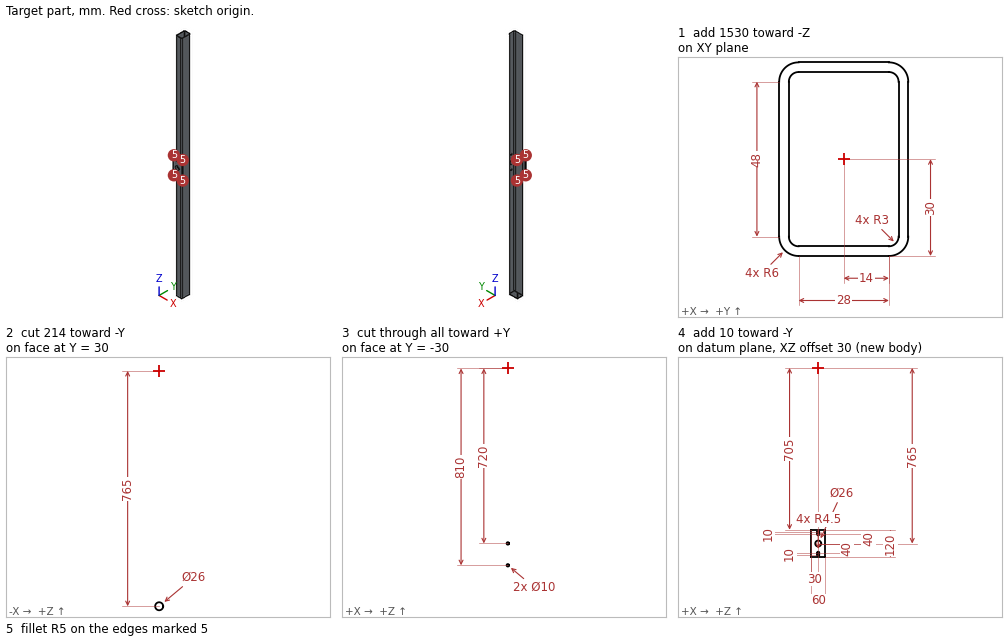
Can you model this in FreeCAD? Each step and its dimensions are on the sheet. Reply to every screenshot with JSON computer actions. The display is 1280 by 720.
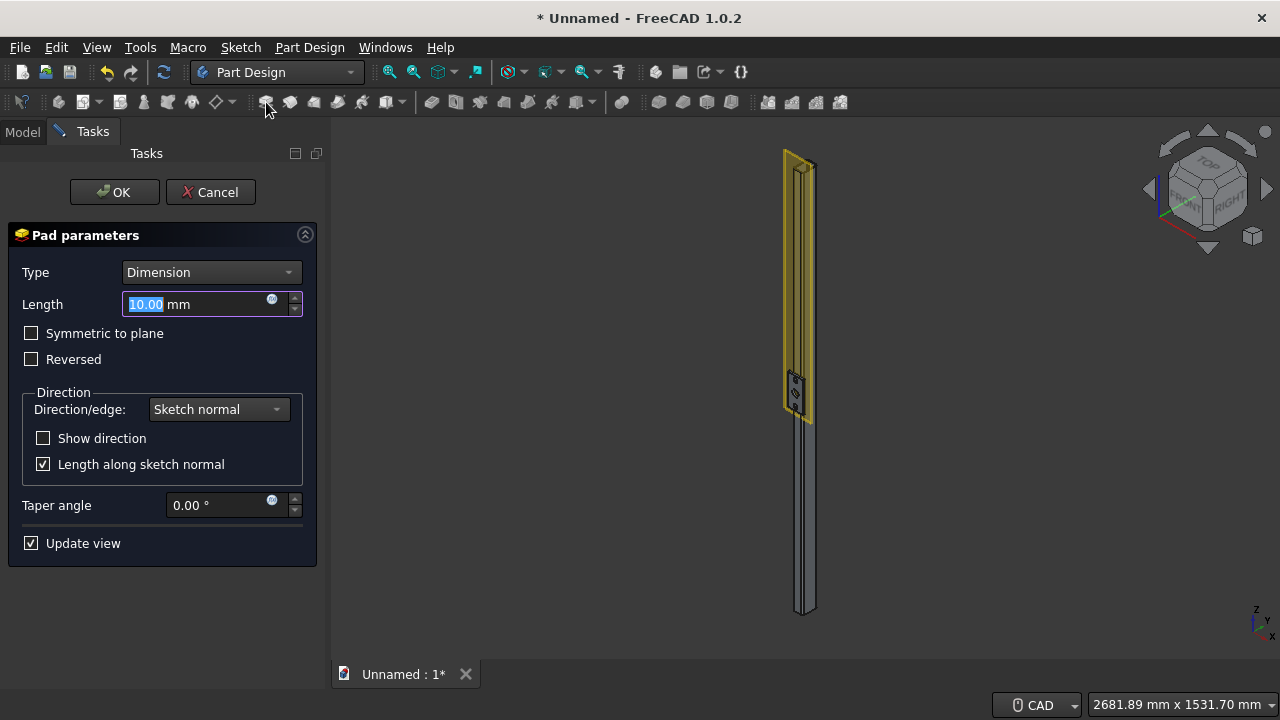
{"action": "type", "text": "10"}
{"action": "key", "text": "Tab"}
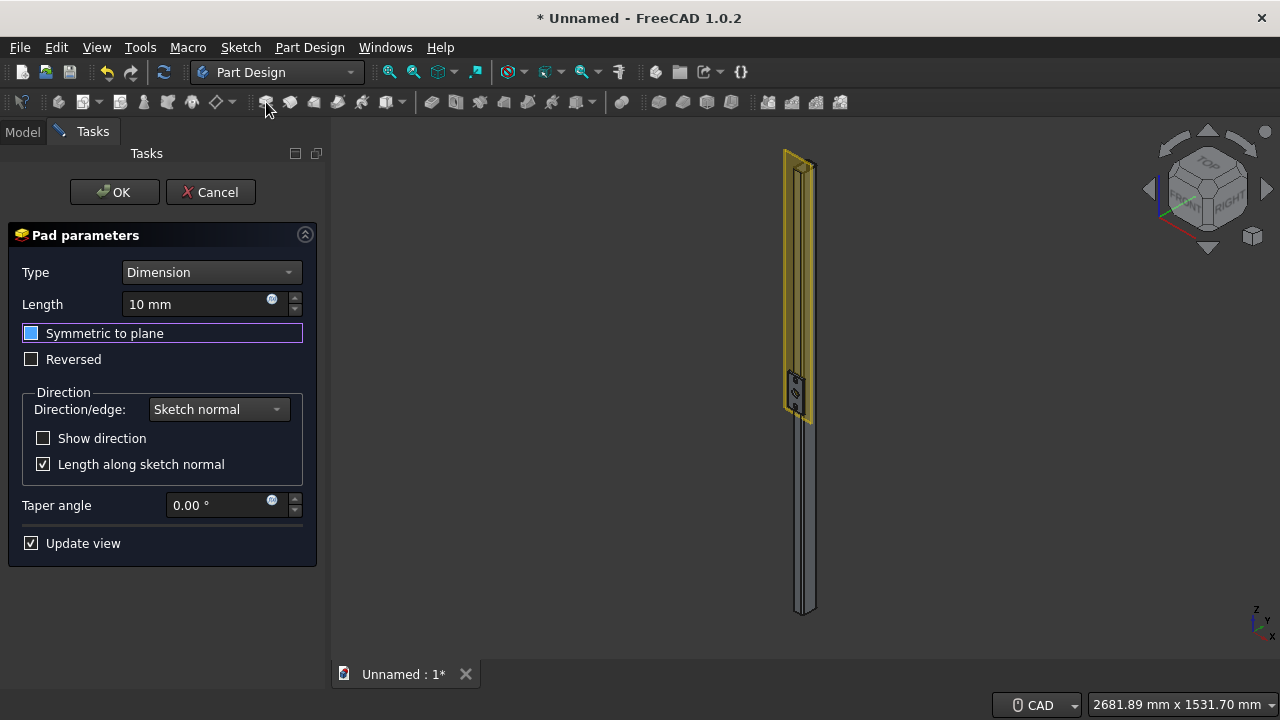
{"action": "left_click", "coordinate": [115, 192]}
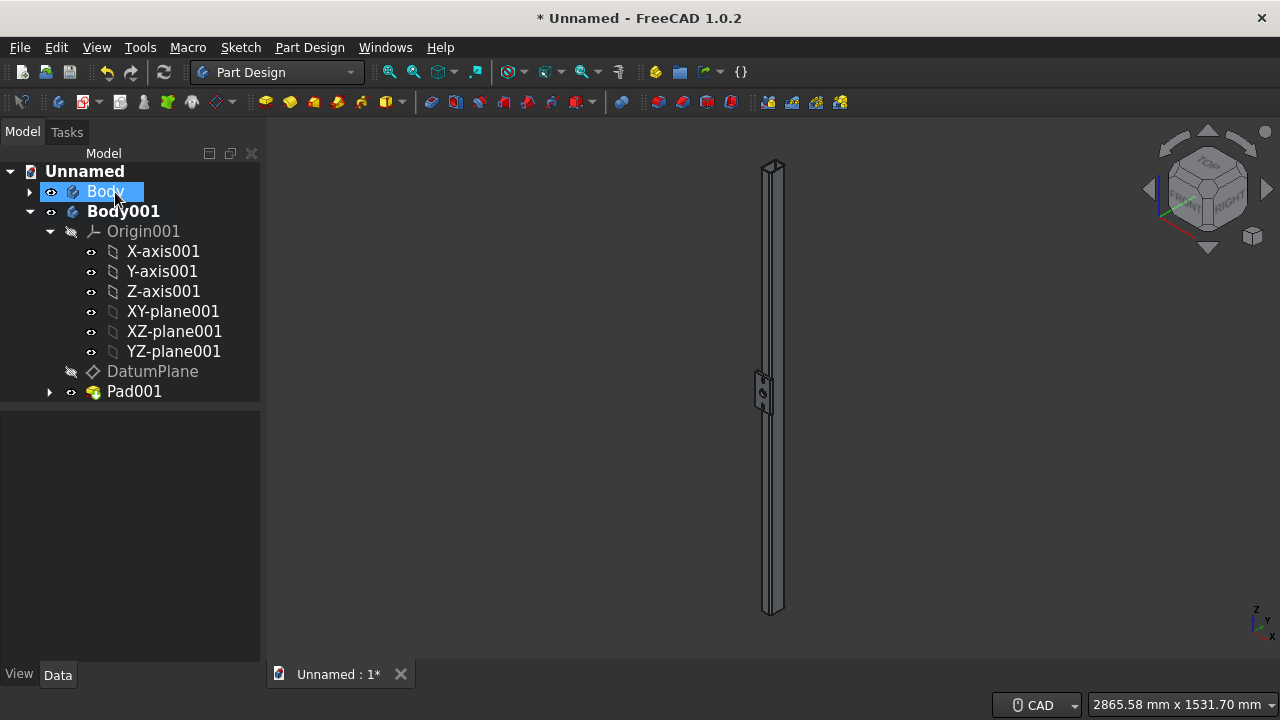
{"action": "left_click", "coordinate": [390, 72]}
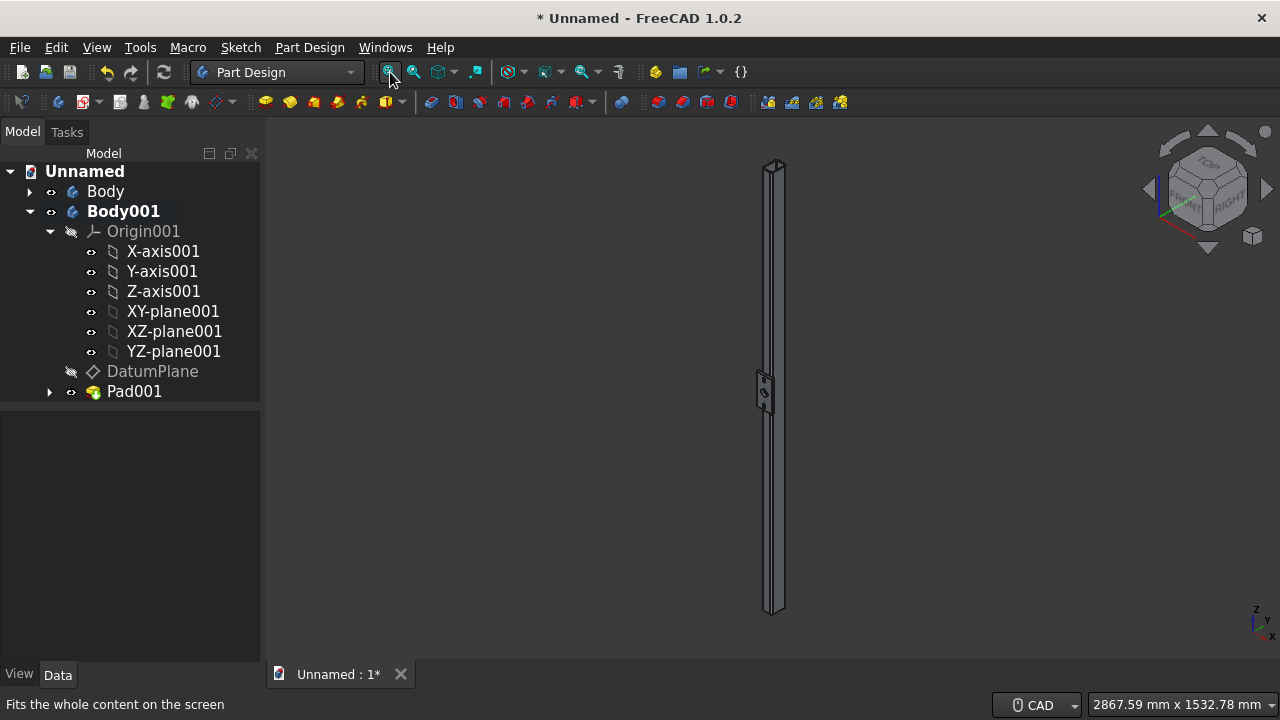
{"action": "scroll", "coordinate": [773, 413], "scroll_direction": "up", "scroll_amount": 13}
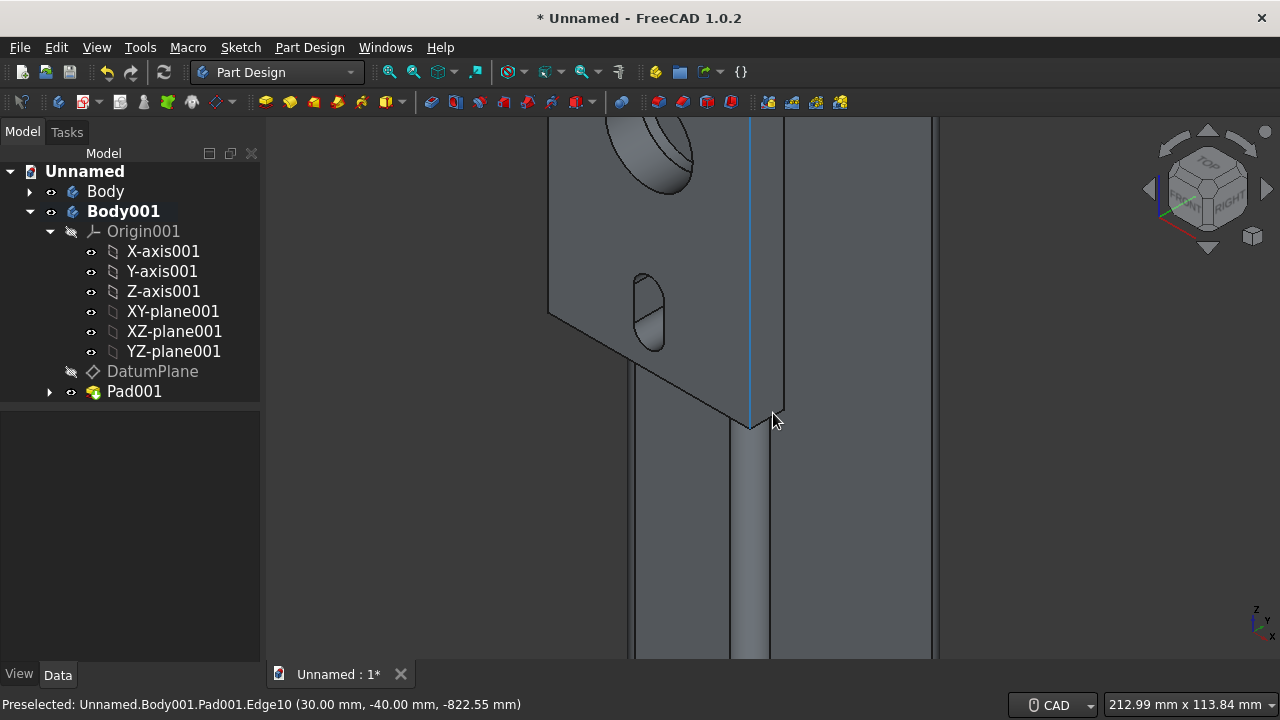
{"action": "left_click", "coordinate": [390, 72]}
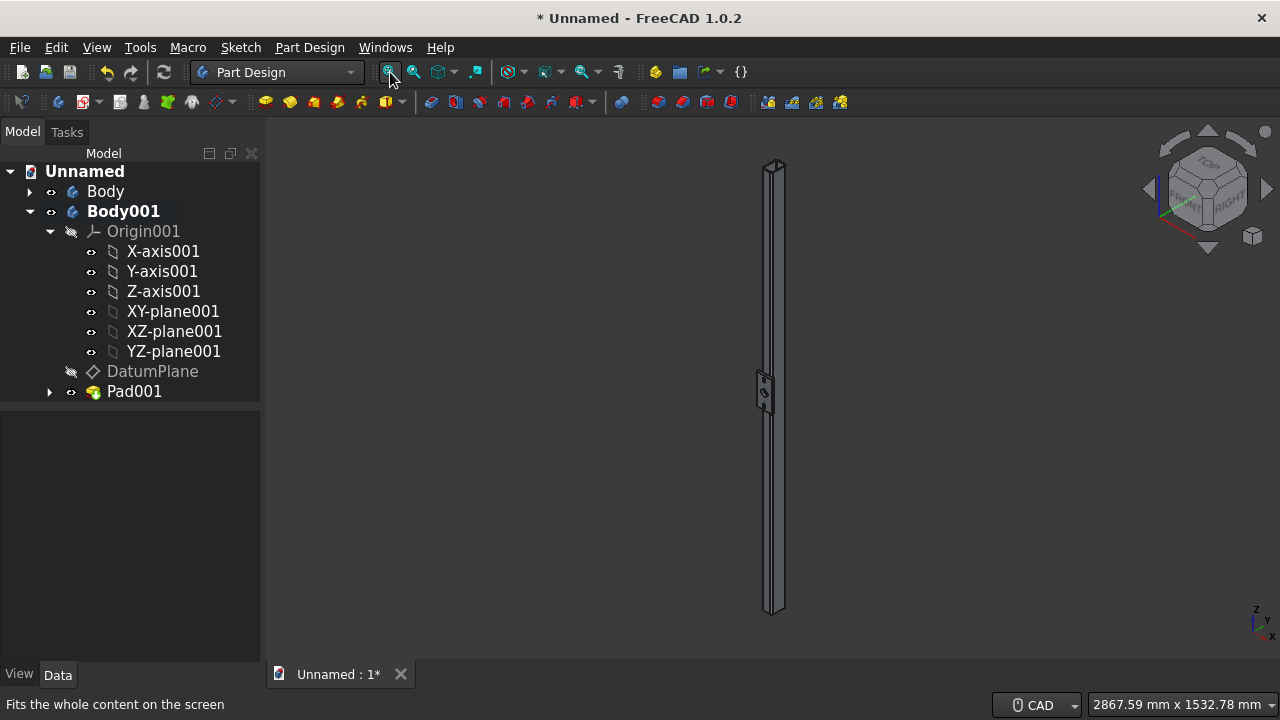
{"action": "key", "text": "2"}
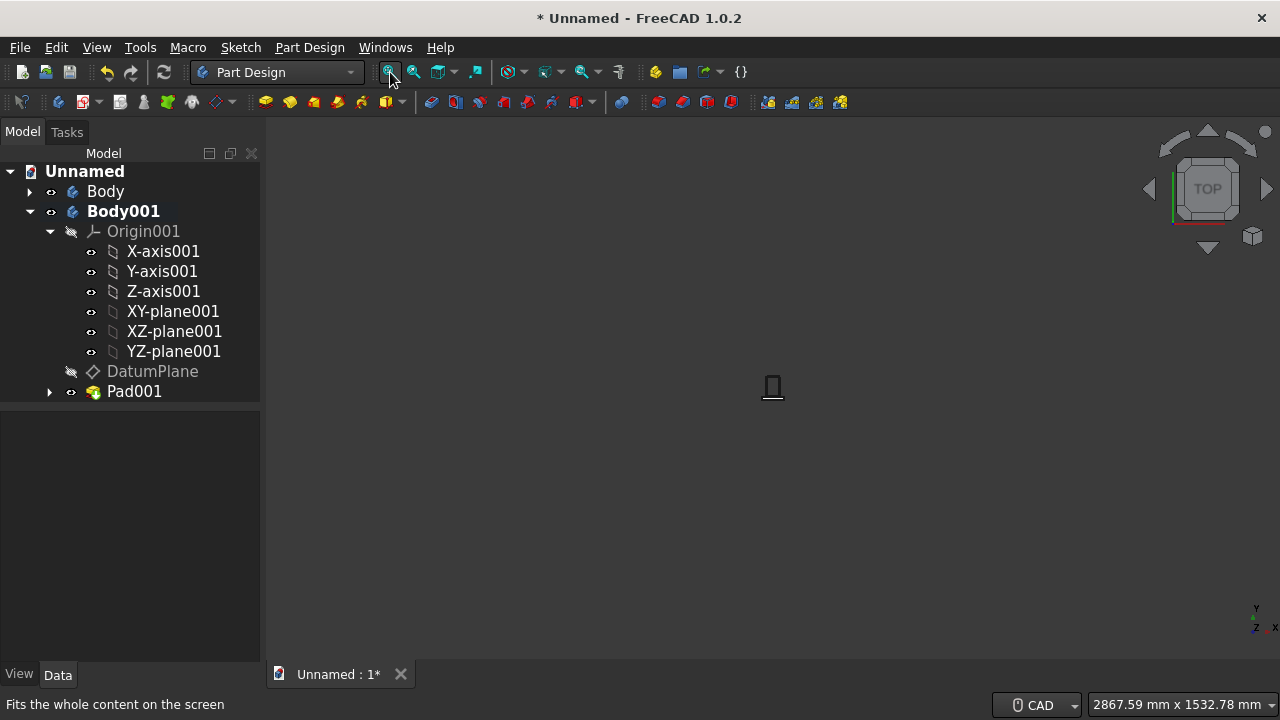
{"action": "left_click", "coordinate": [390, 72]}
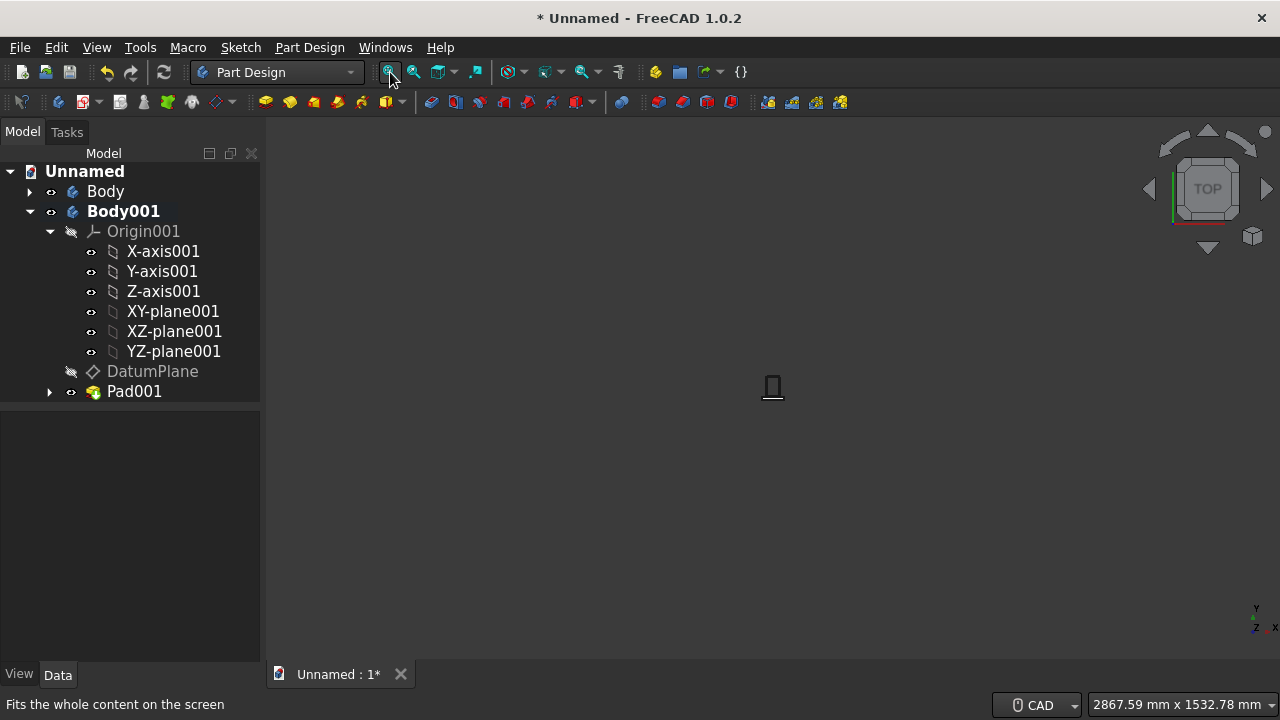
{"action": "scroll", "coordinate": [784, 398], "scroll_direction": "up", "scroll_amount": 13}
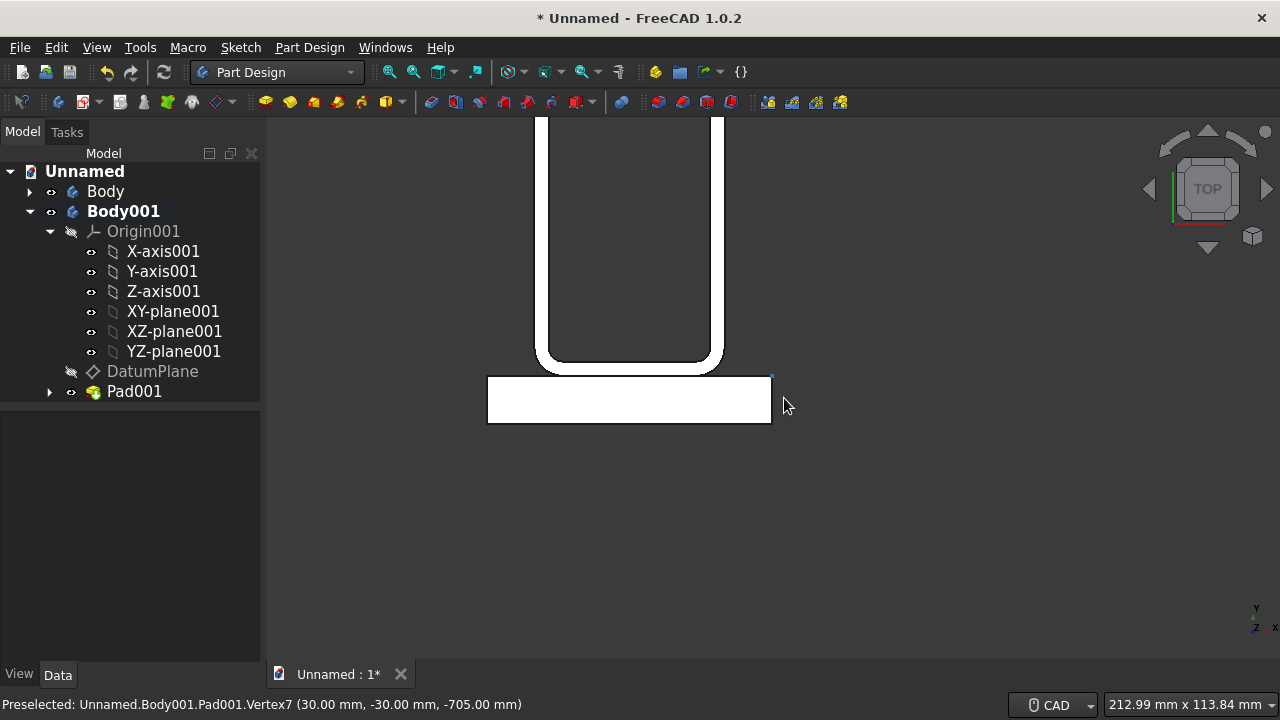
{"action": "left_click", "coordinate": [487, 399]}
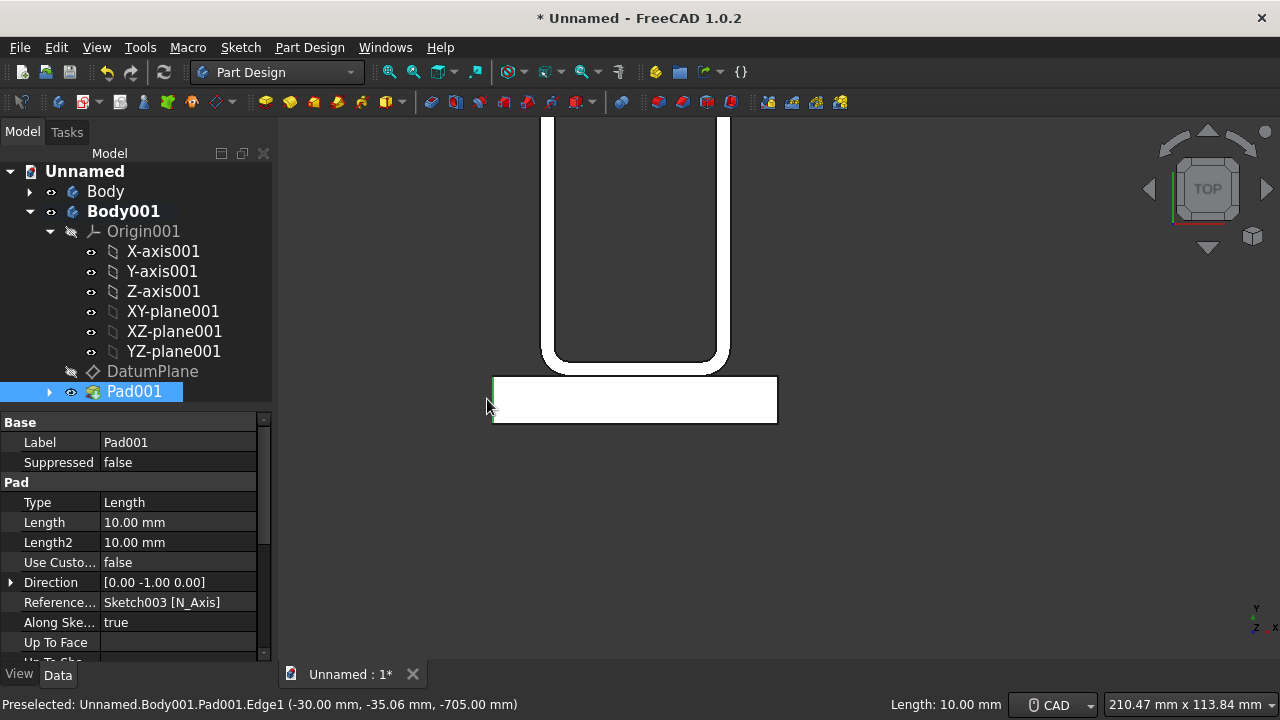
{"action": "left_click", "coordinate": [778, 399], "text": "ctrl"}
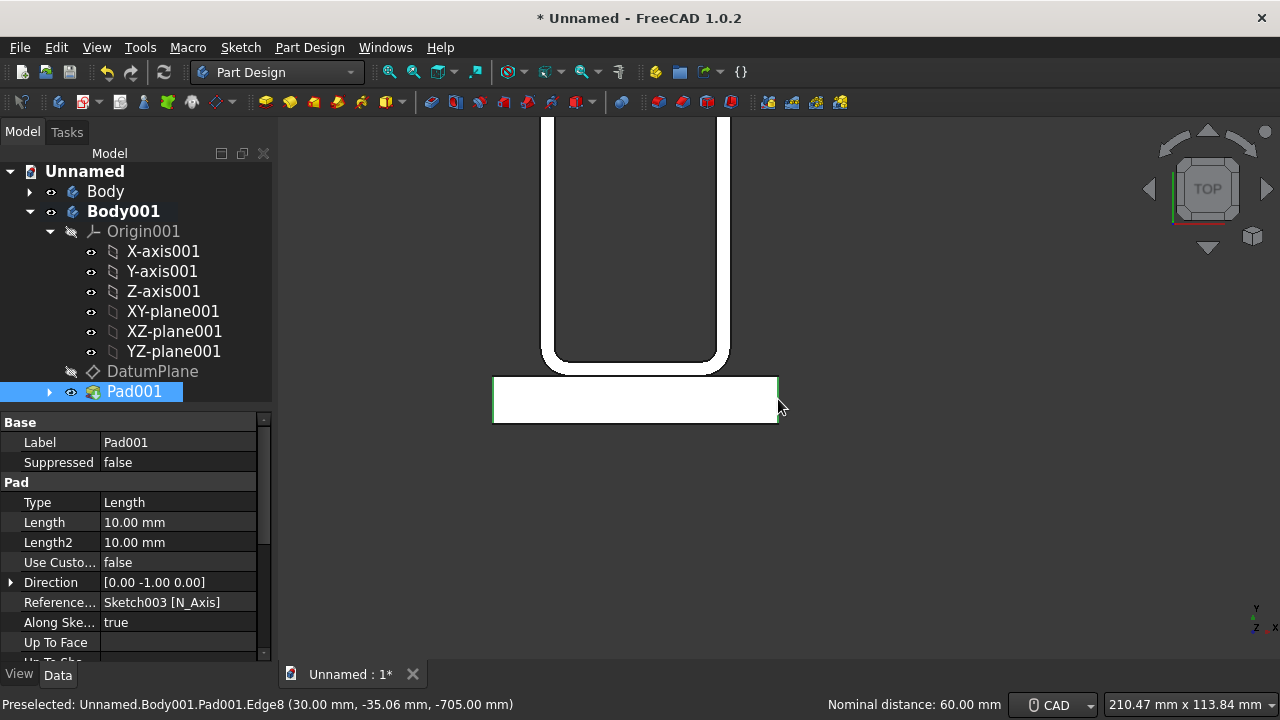
{"action": "left_click", "coordinate": [390, 72]}